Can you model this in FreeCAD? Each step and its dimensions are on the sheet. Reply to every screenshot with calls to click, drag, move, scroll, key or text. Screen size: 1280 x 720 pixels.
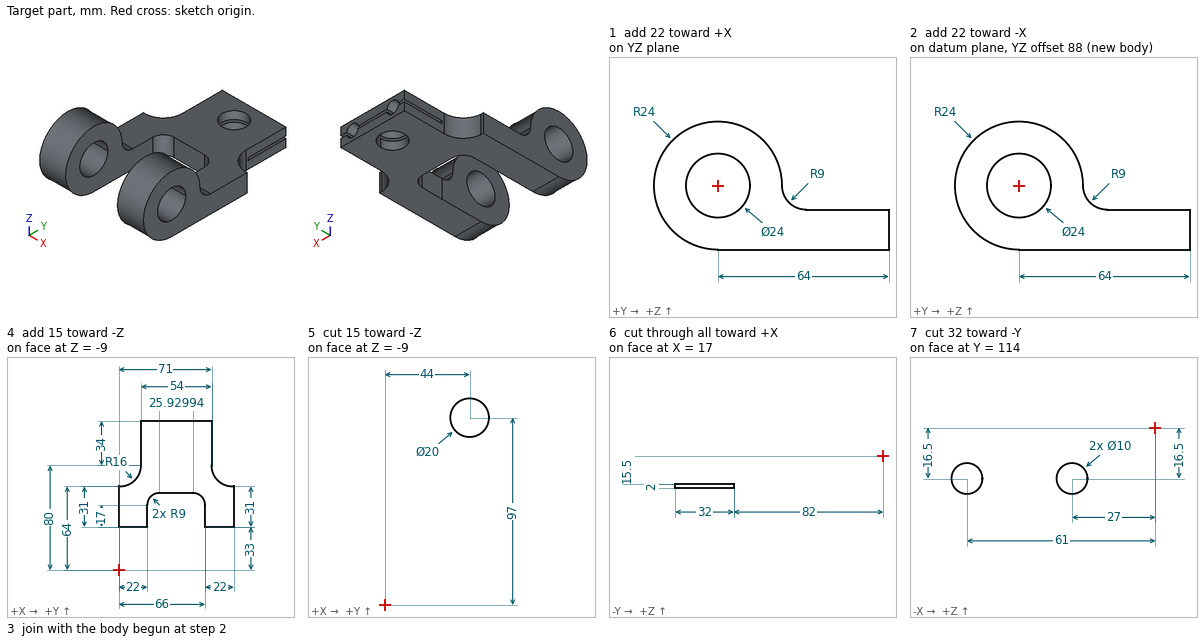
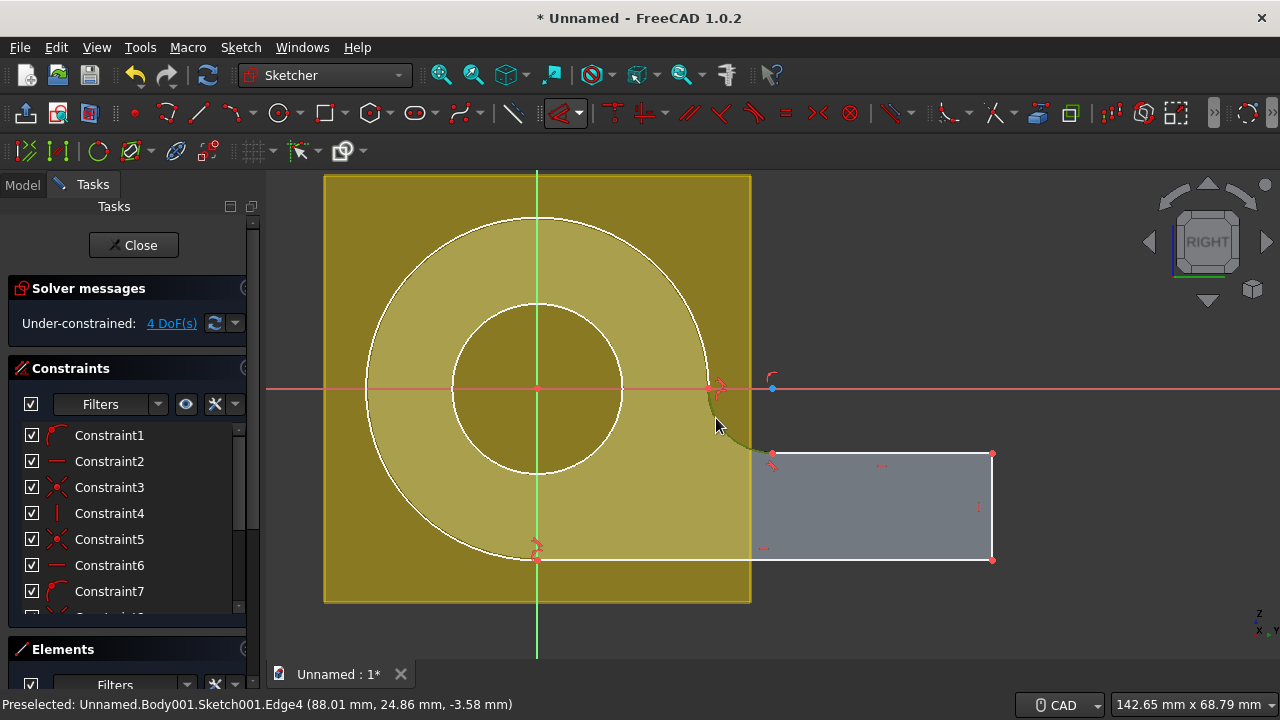
key(k)
key(r)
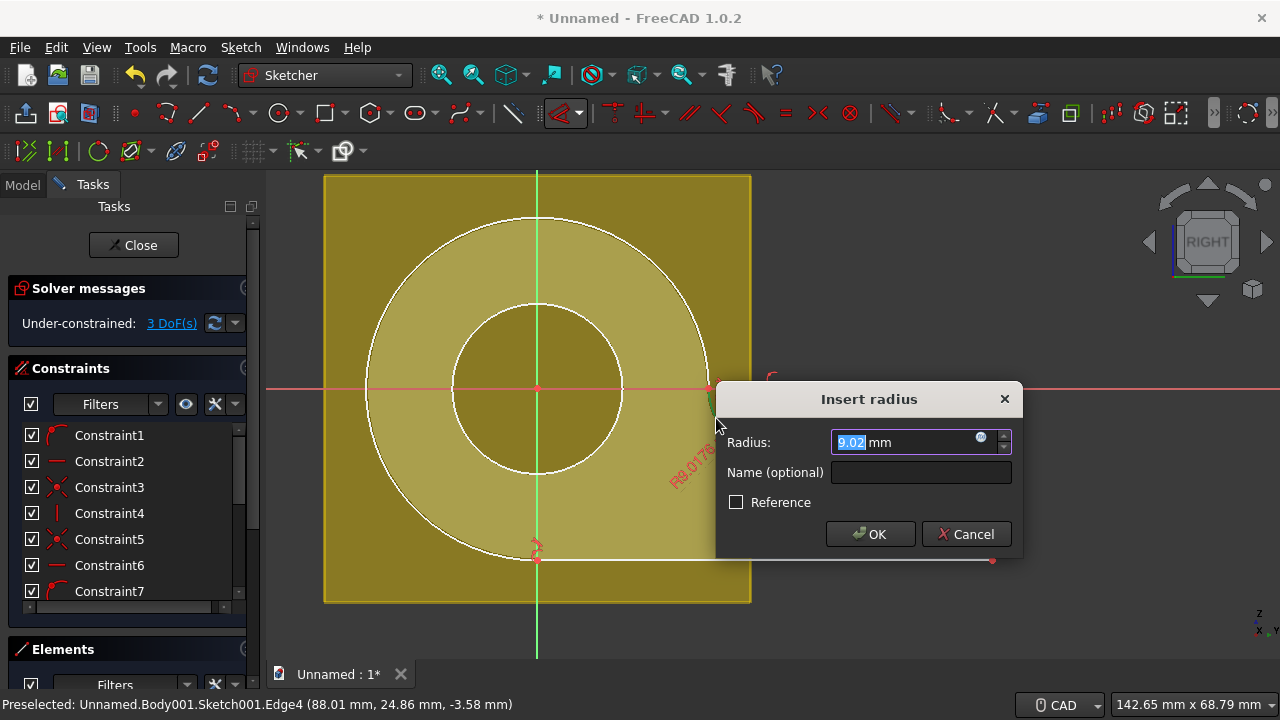
text(9)
key(Return)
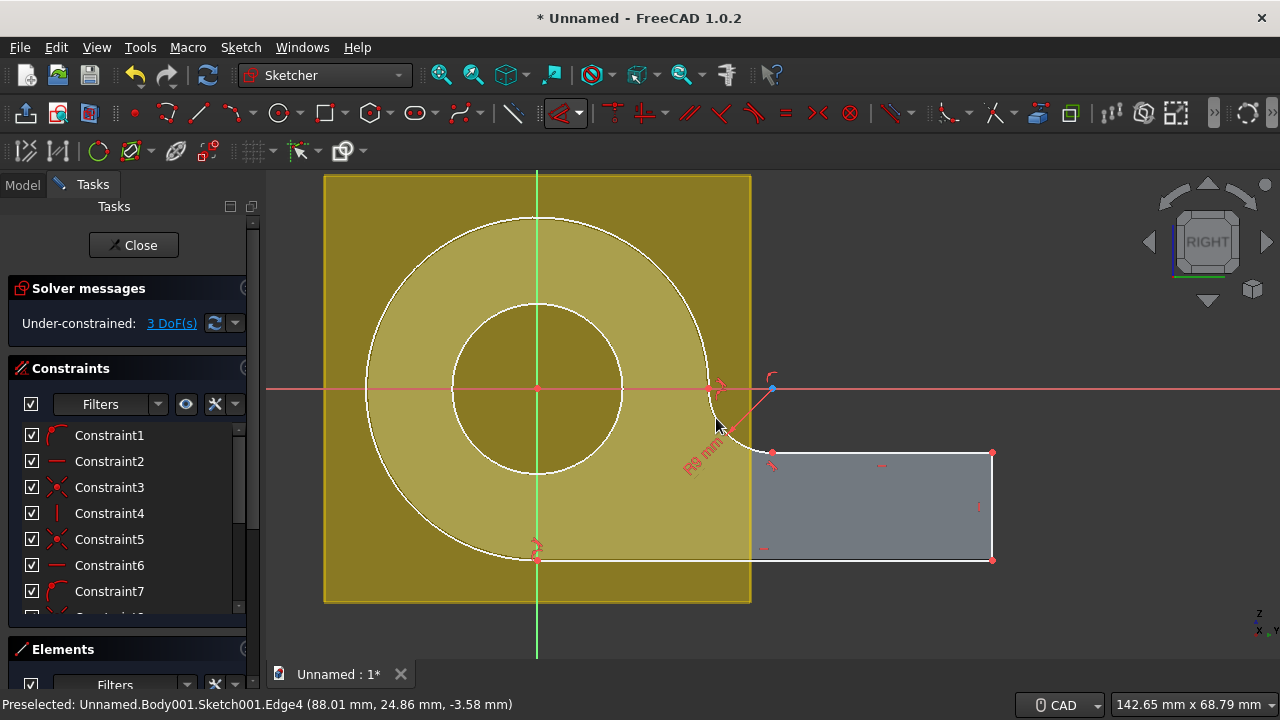
click(564, 220)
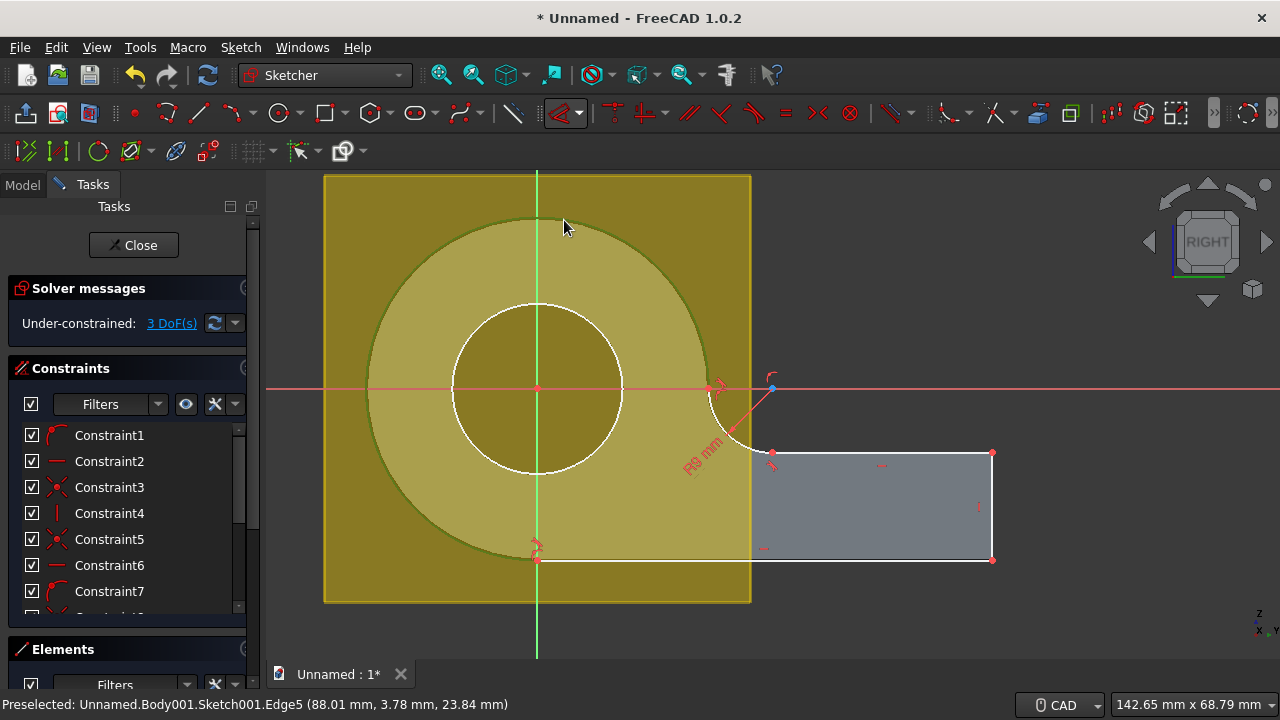
click(582, 114)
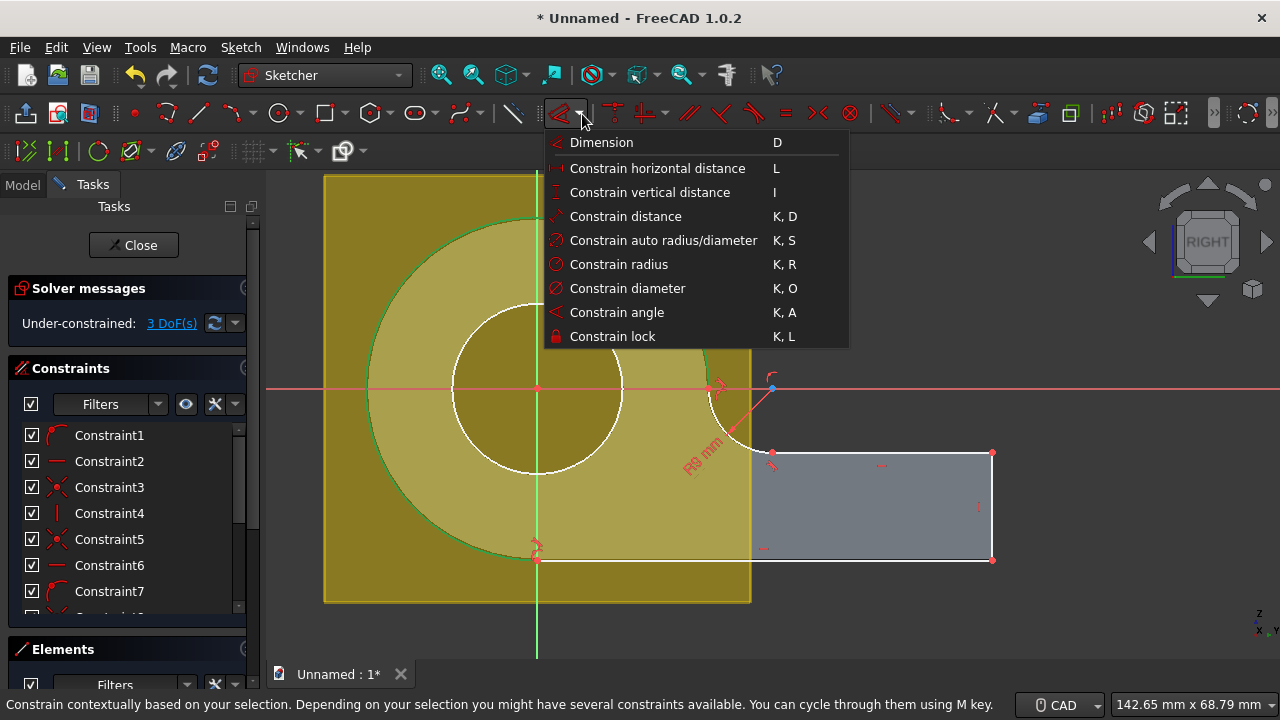
click(697, 264)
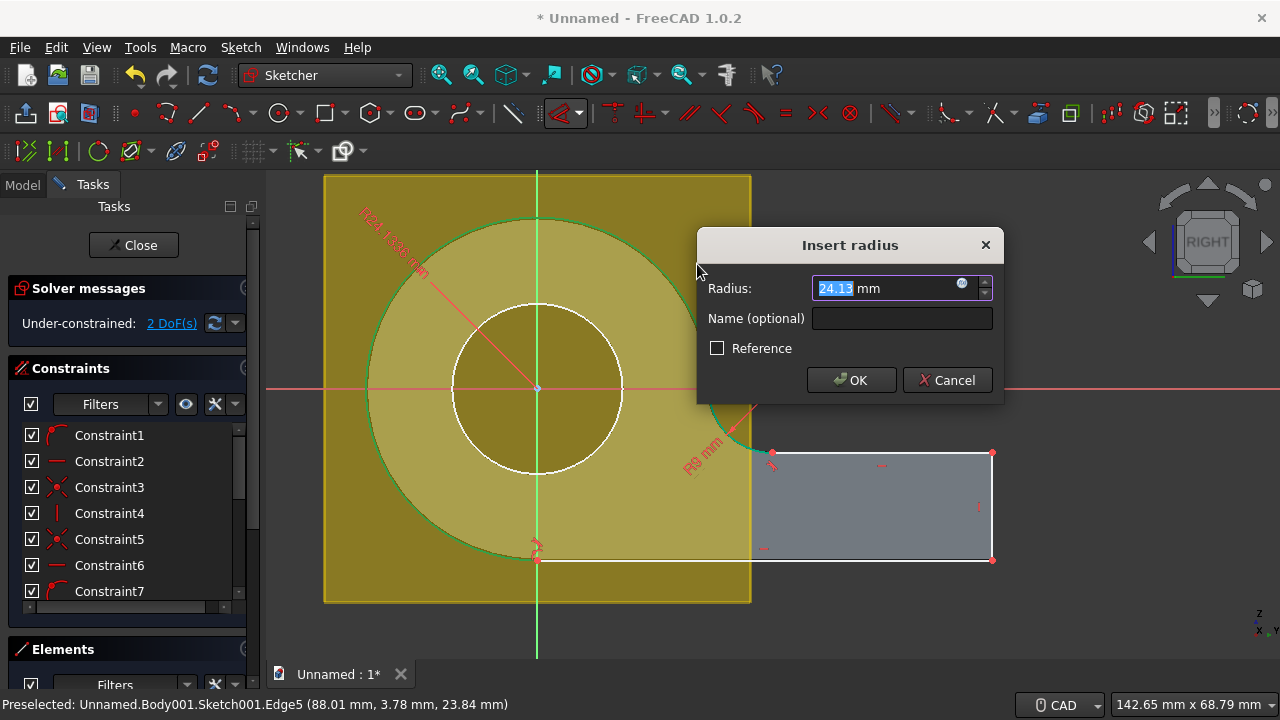
text(24)
key(Return)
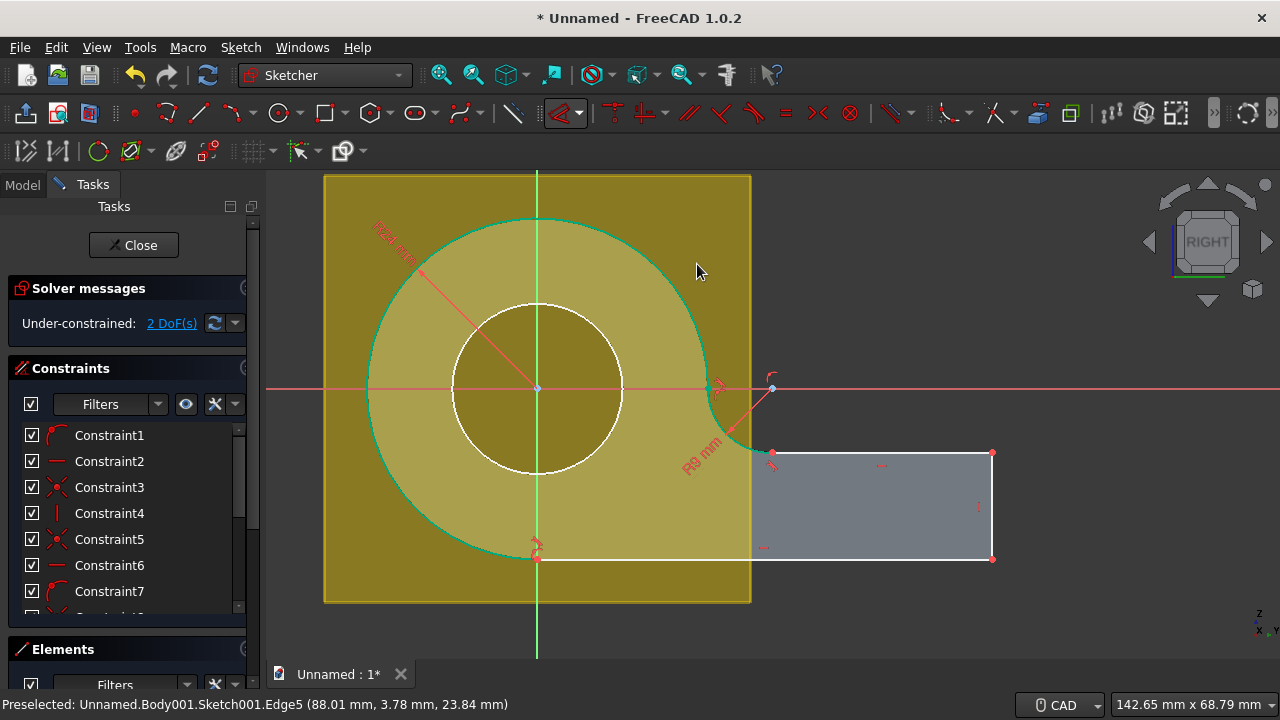
click(597, 329)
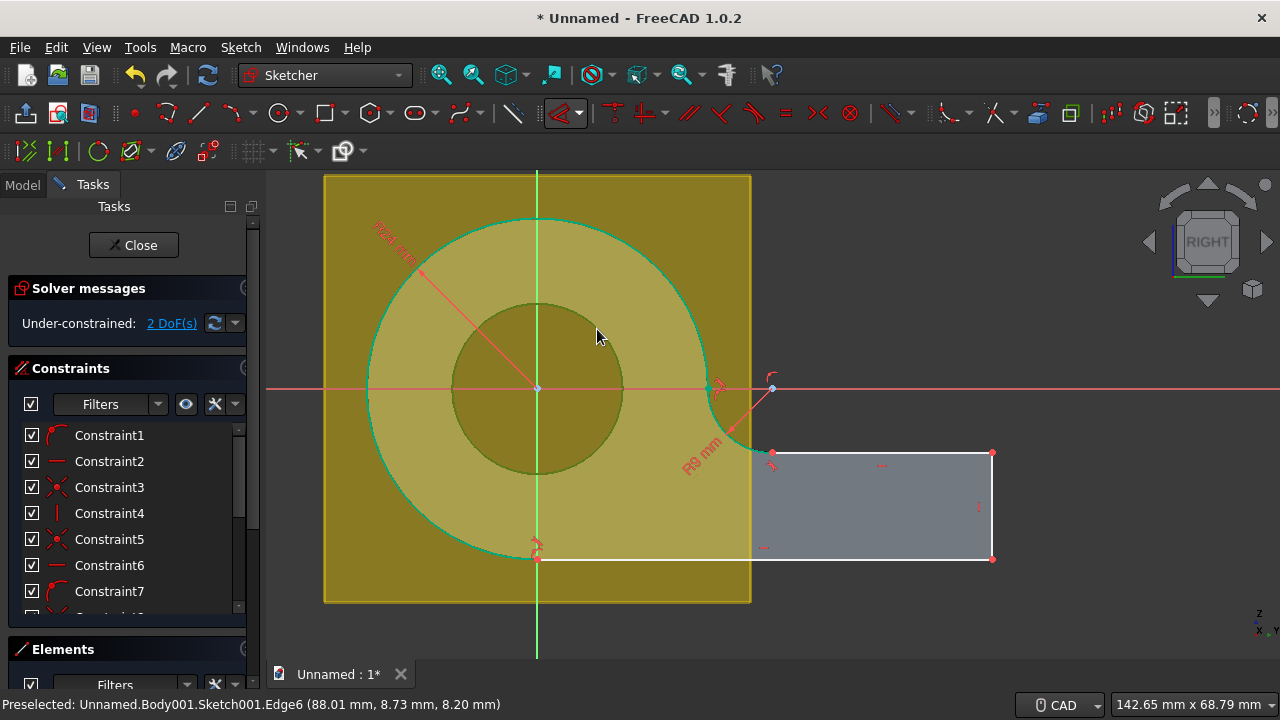
key(k)
key(o)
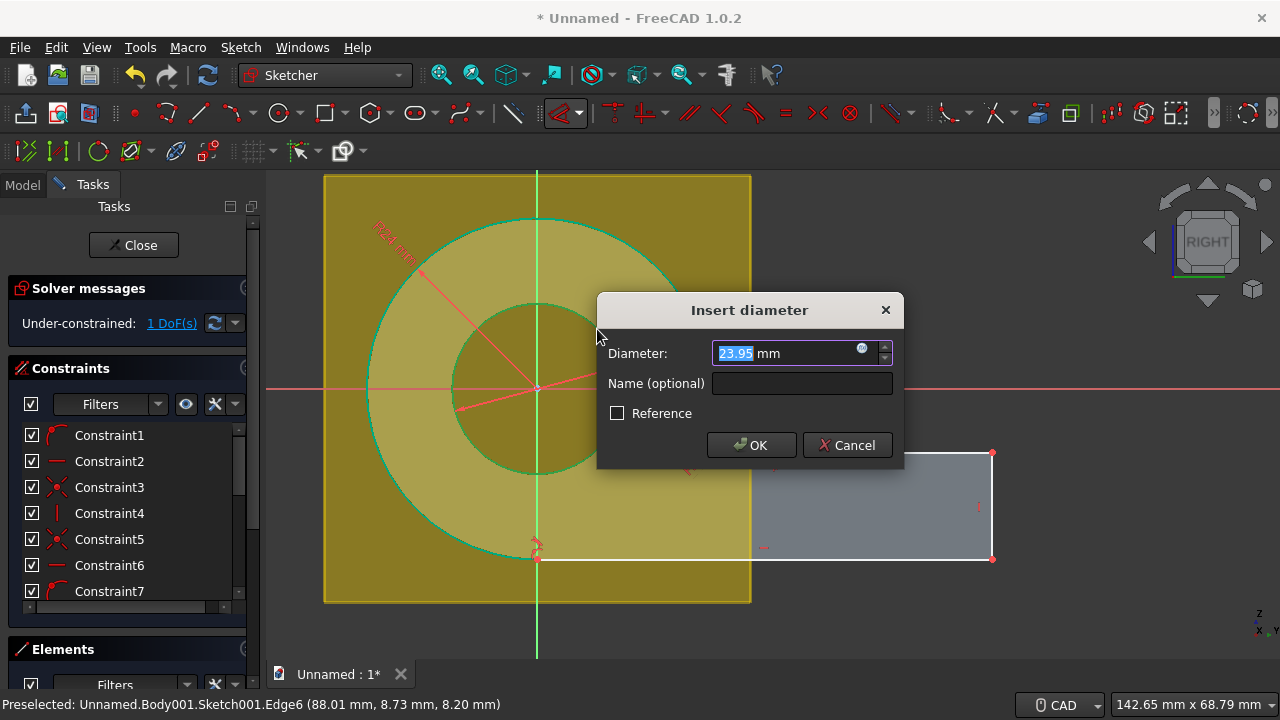
text(24)
key(Return)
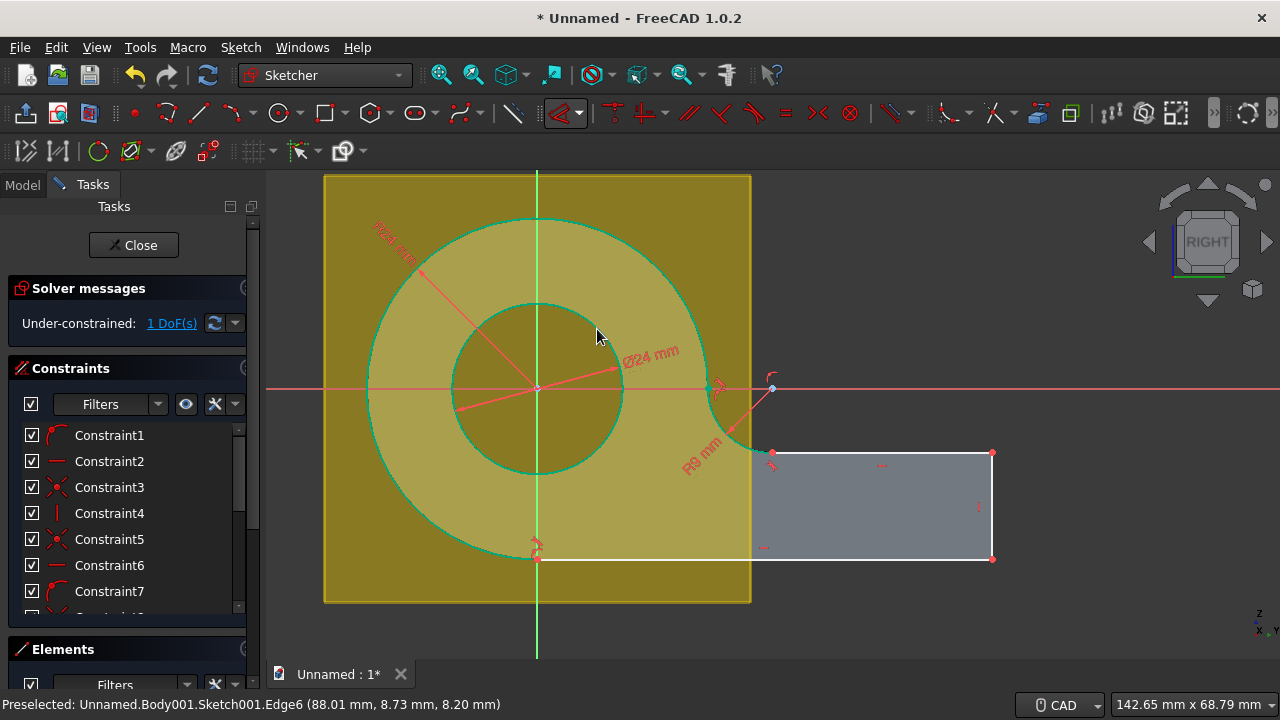
click(674, 560)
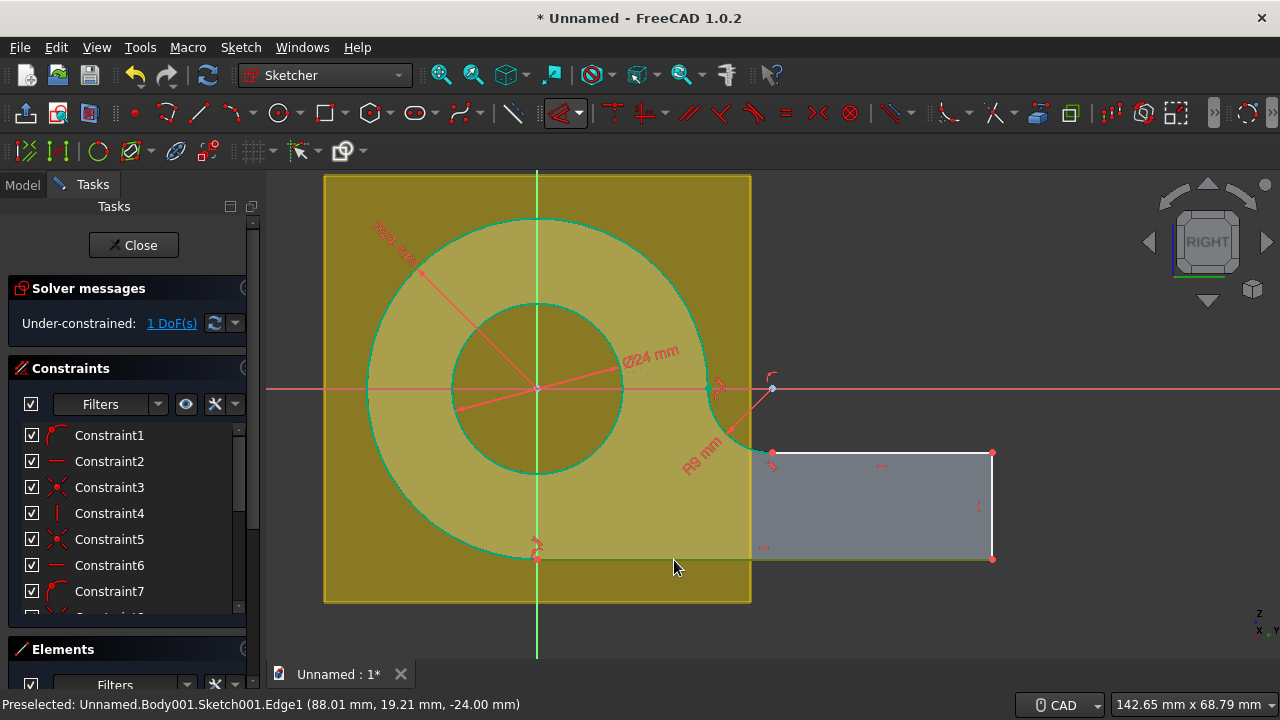
click(582, 114)